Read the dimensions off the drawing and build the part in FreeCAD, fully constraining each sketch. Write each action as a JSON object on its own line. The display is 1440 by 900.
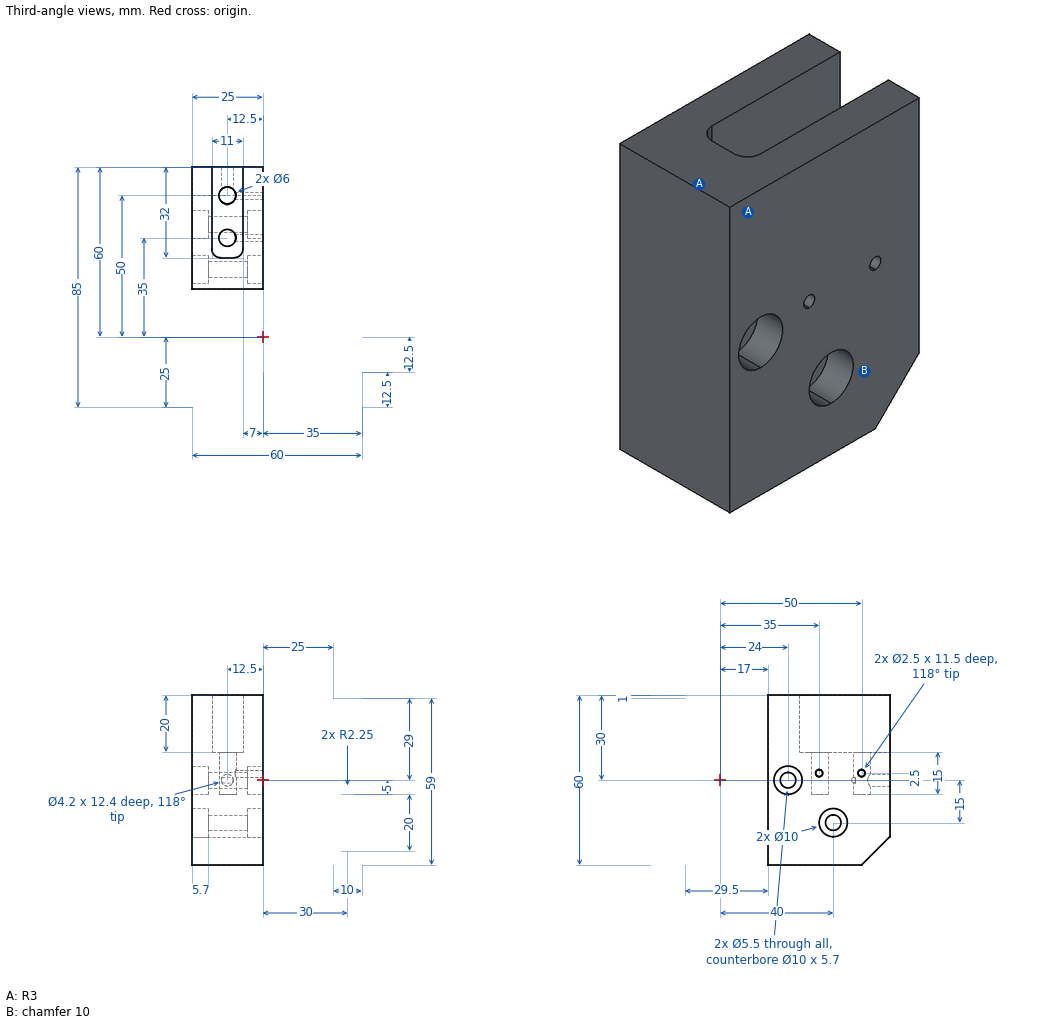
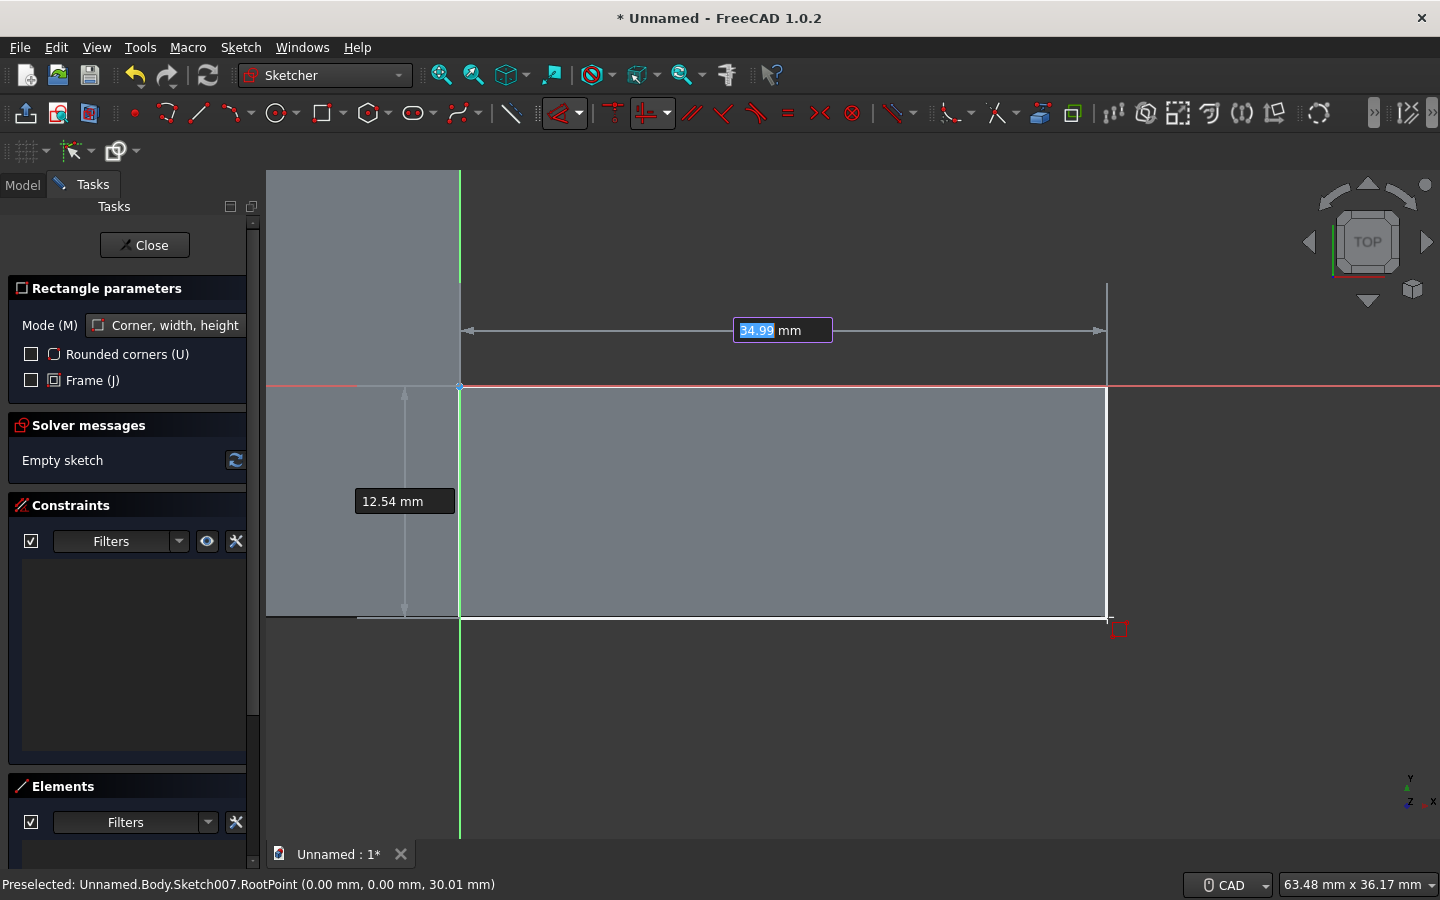
{"action": "type", "text": "35"}
{"action": "key", "text": "Tab"}
{"action": "type", "text": "12.5"}
{"action": "key", "text": "Return"}
{"action": "key", "text": "Escape"}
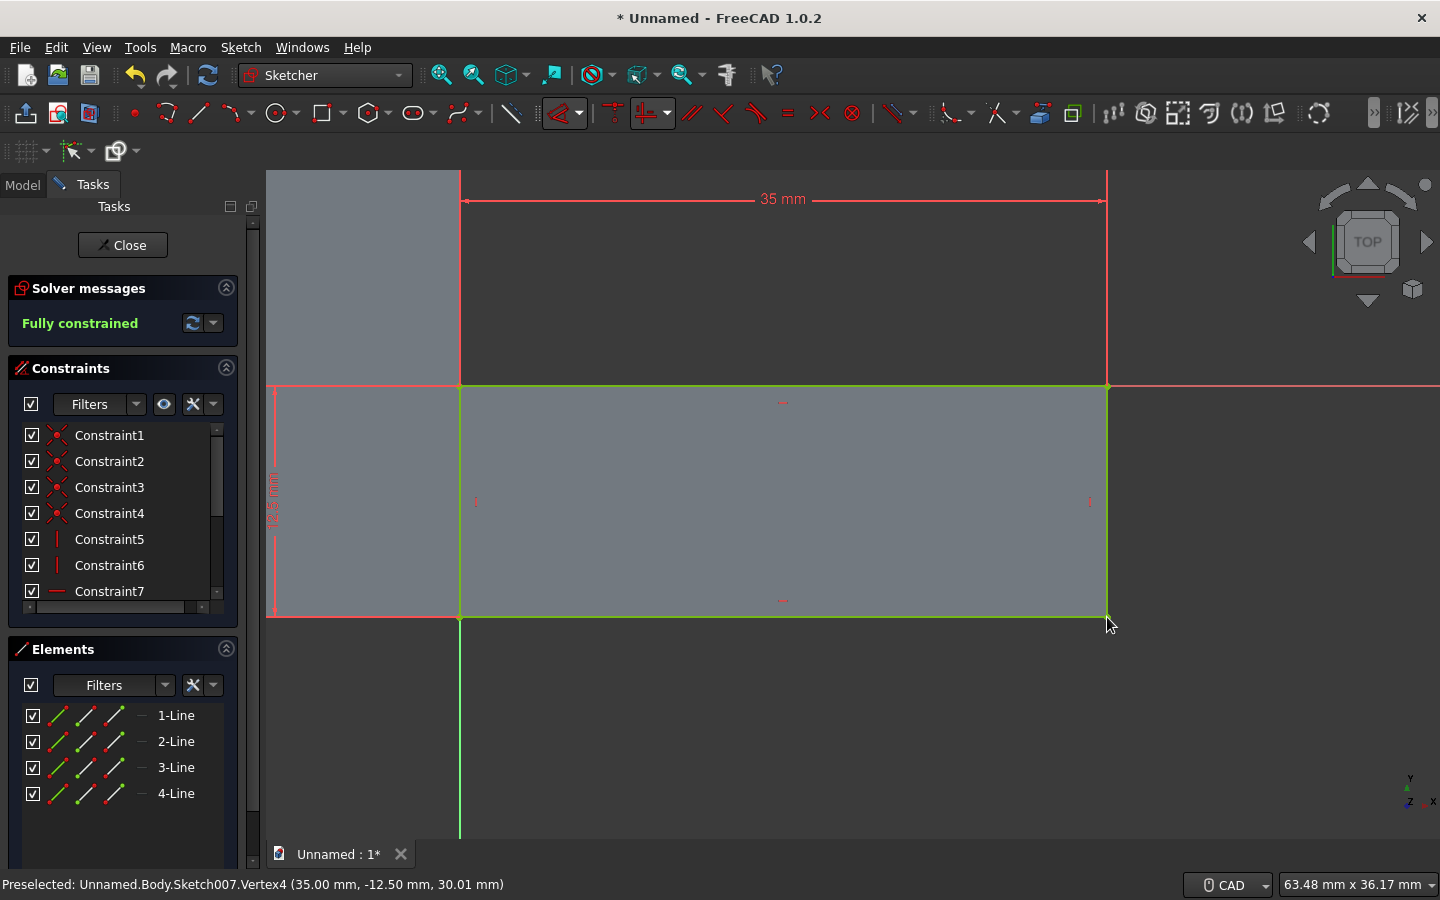
{"action": "left_click", "coordinate": [123, 245]}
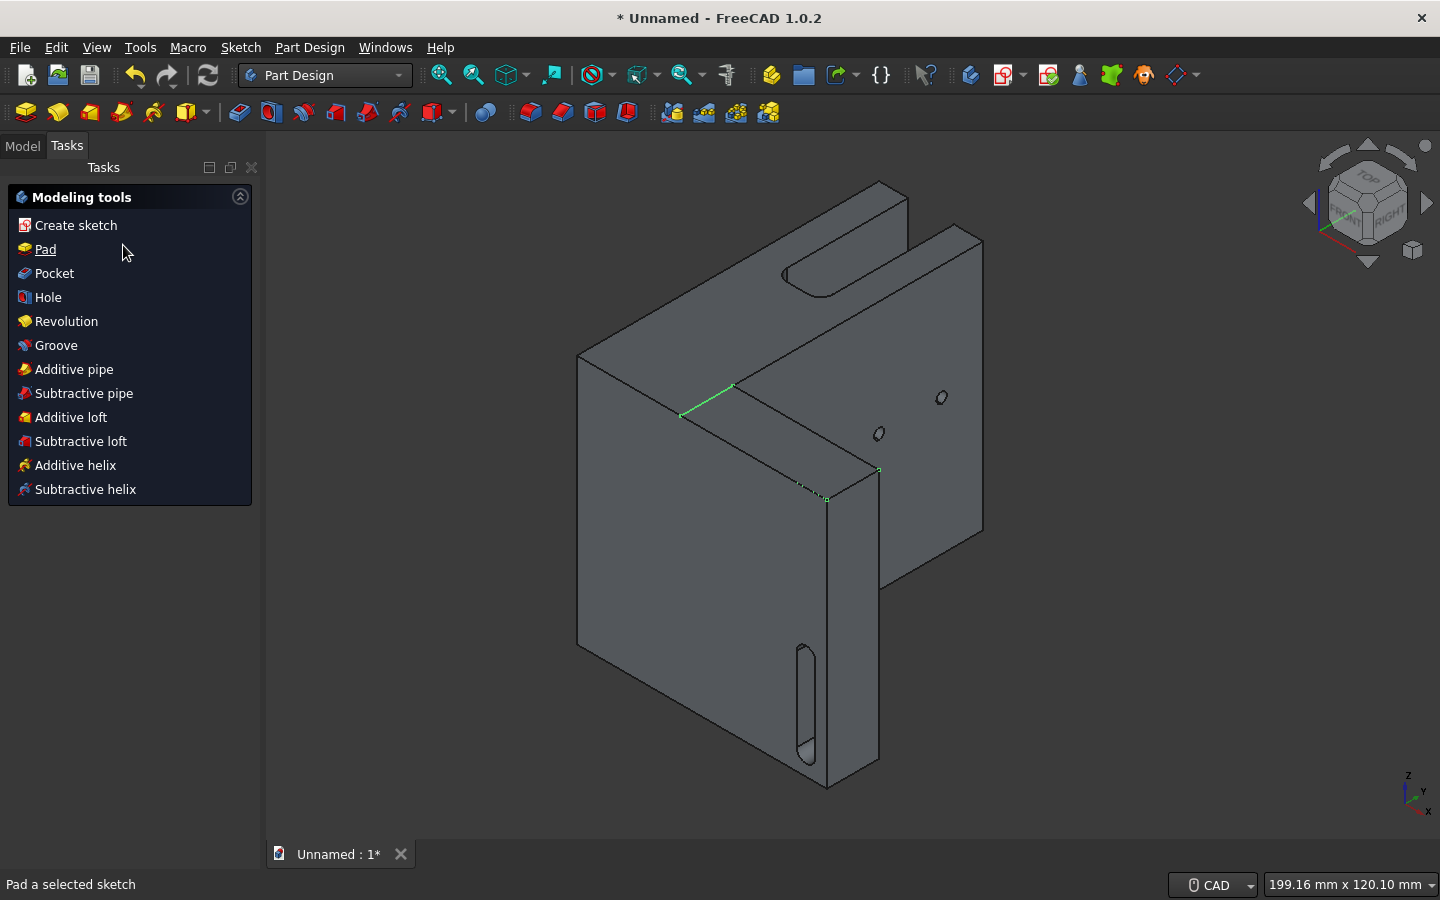
{"action": "left_click", "coordinate": [240, 112]}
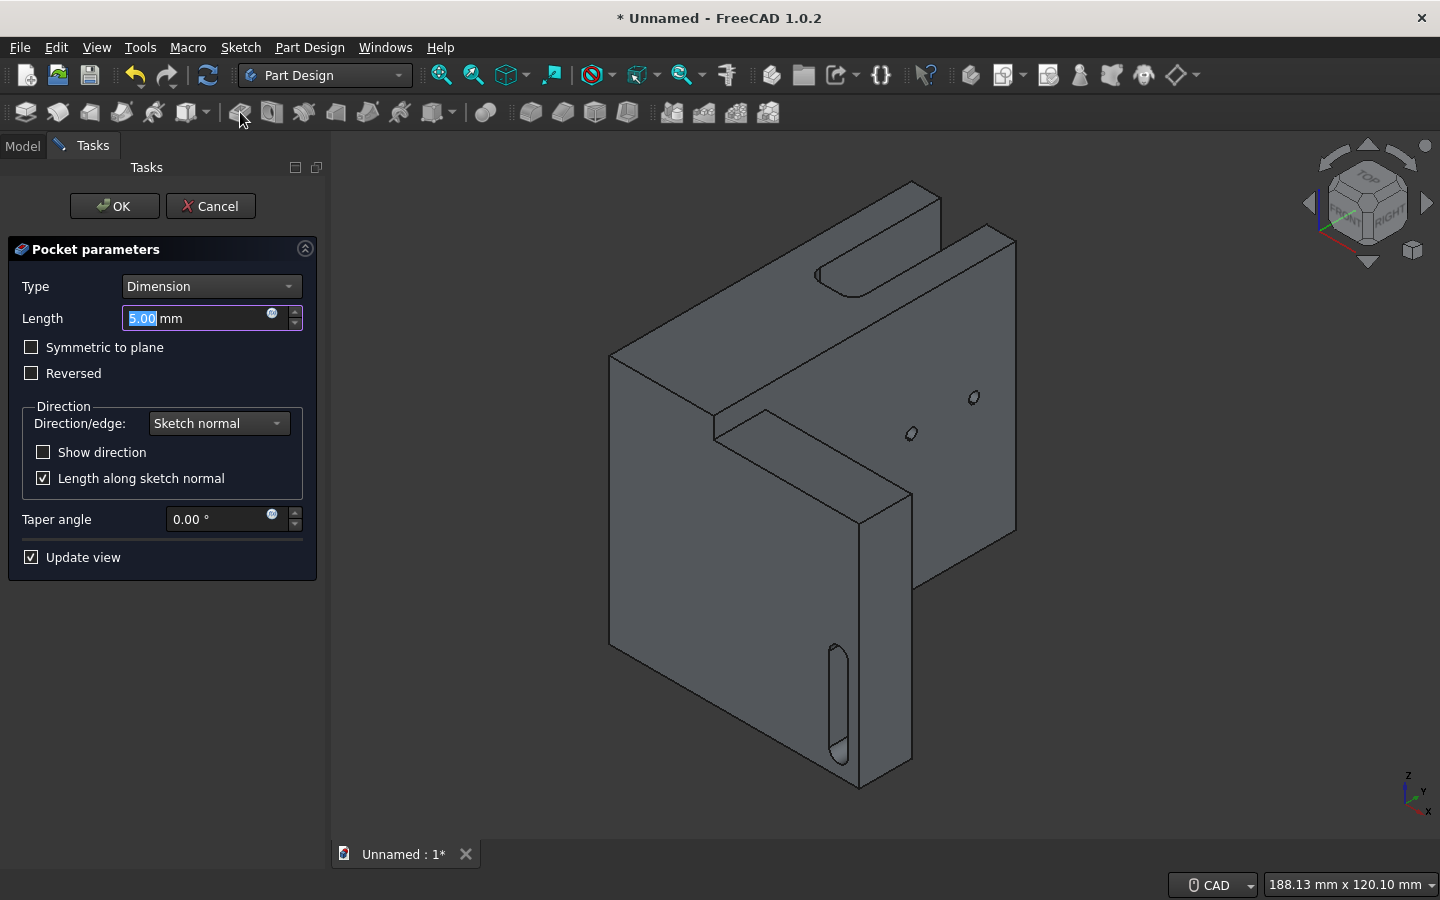
{"action": "type", "text": "1"}
{"action": "key", "text": "Tab"}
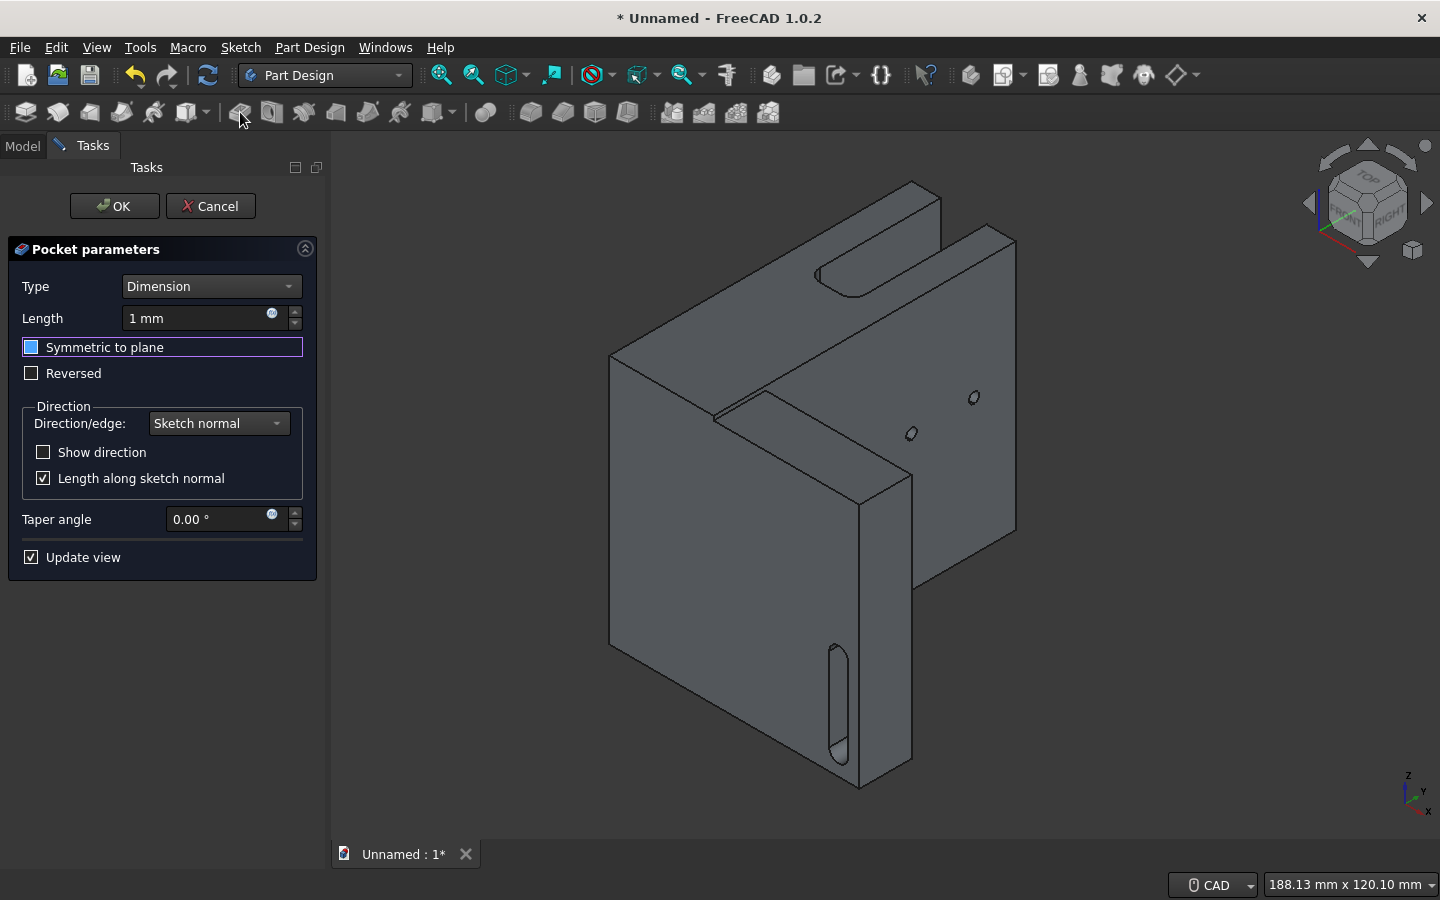
{"action": "left_click", "coordinate": [115, 206]}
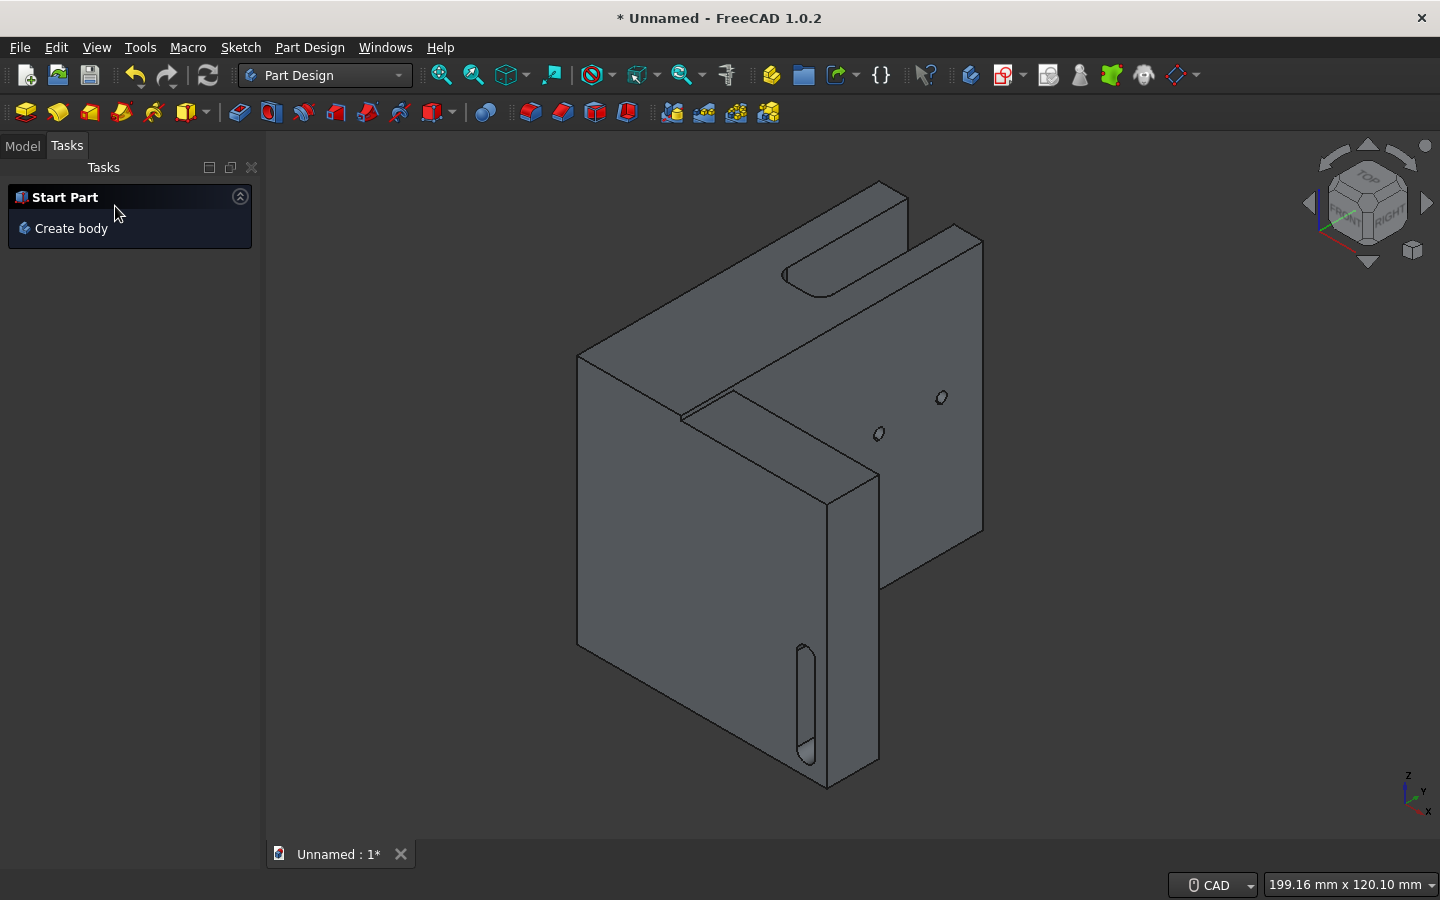
{"action": "left_click", "coordinate": [1004, 76]}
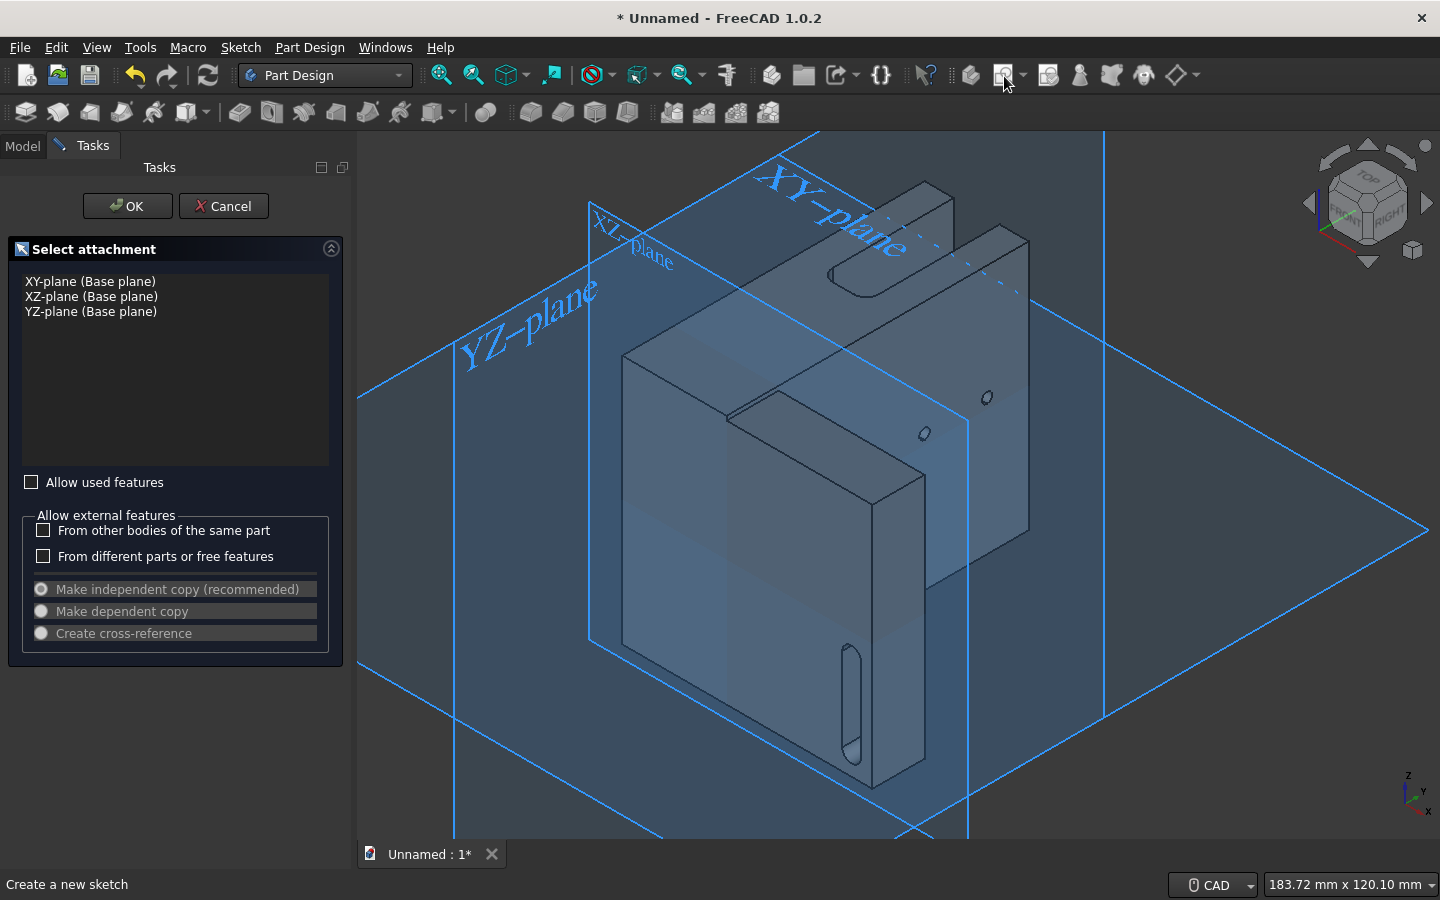
{"action": "left_click", "coordinate": [82, 296]}